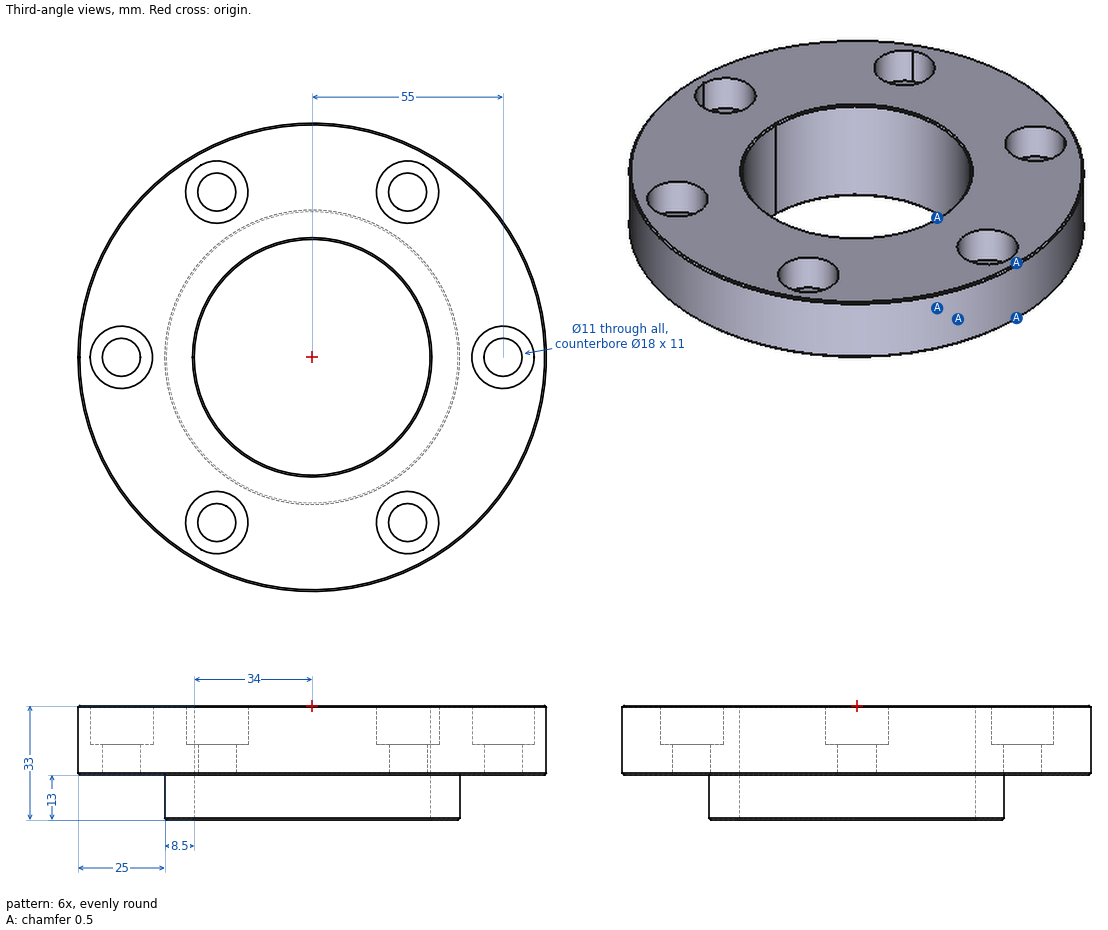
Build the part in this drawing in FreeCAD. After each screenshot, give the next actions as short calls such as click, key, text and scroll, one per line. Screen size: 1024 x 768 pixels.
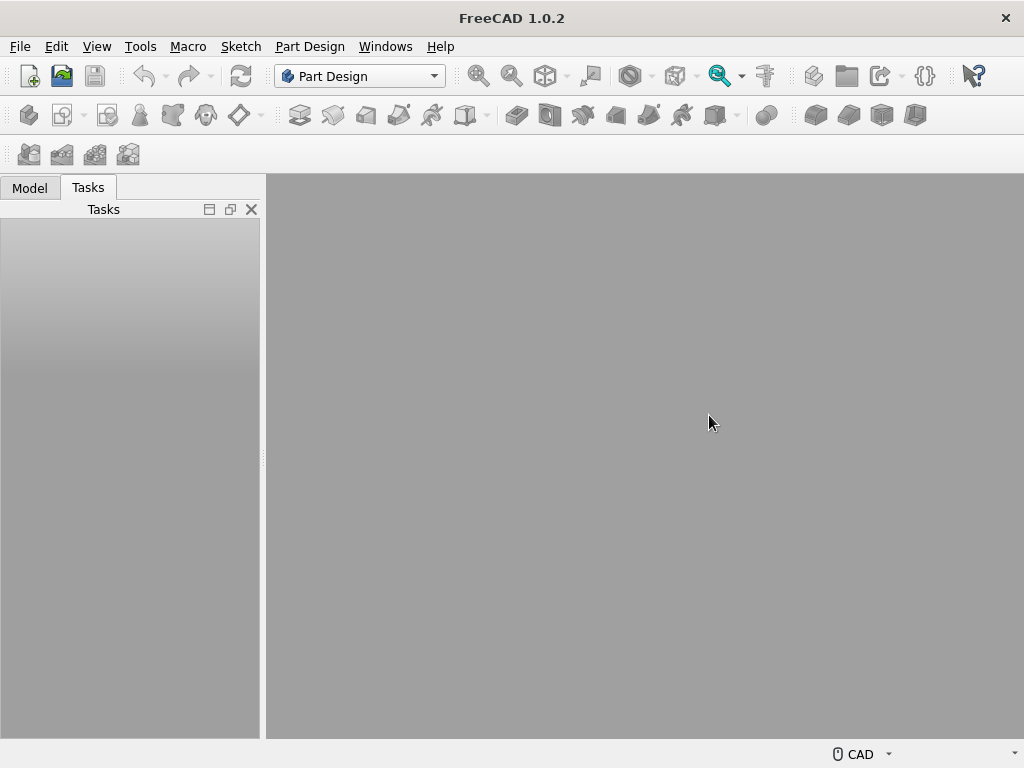
click(29, 76)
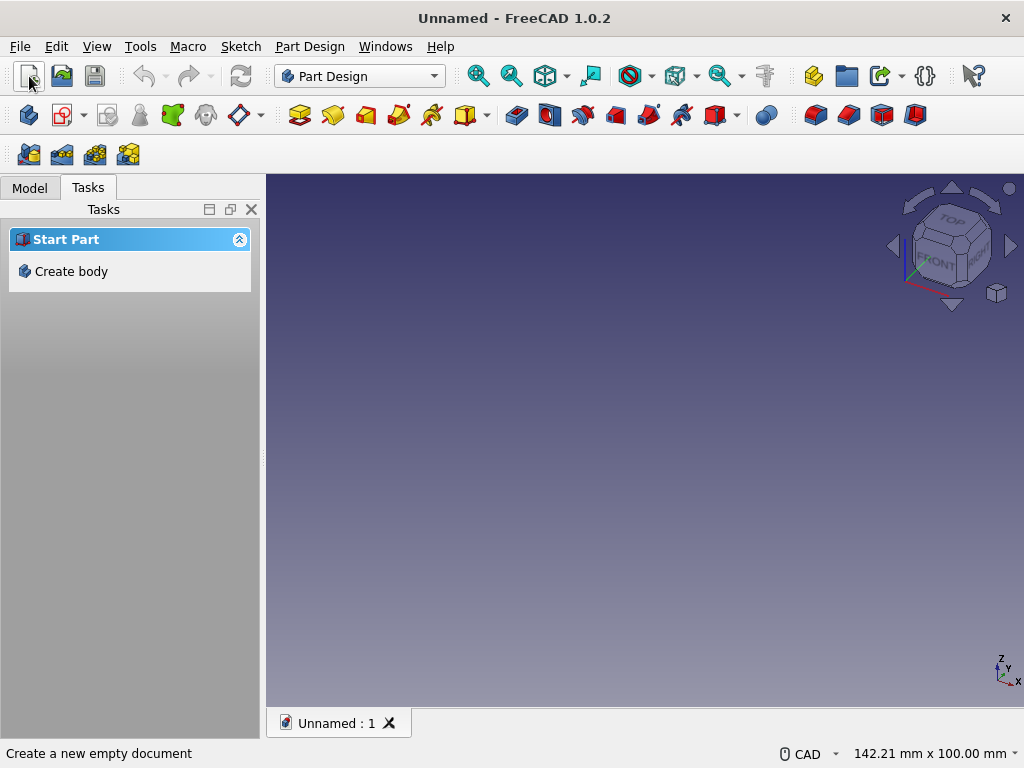
click(62, 116)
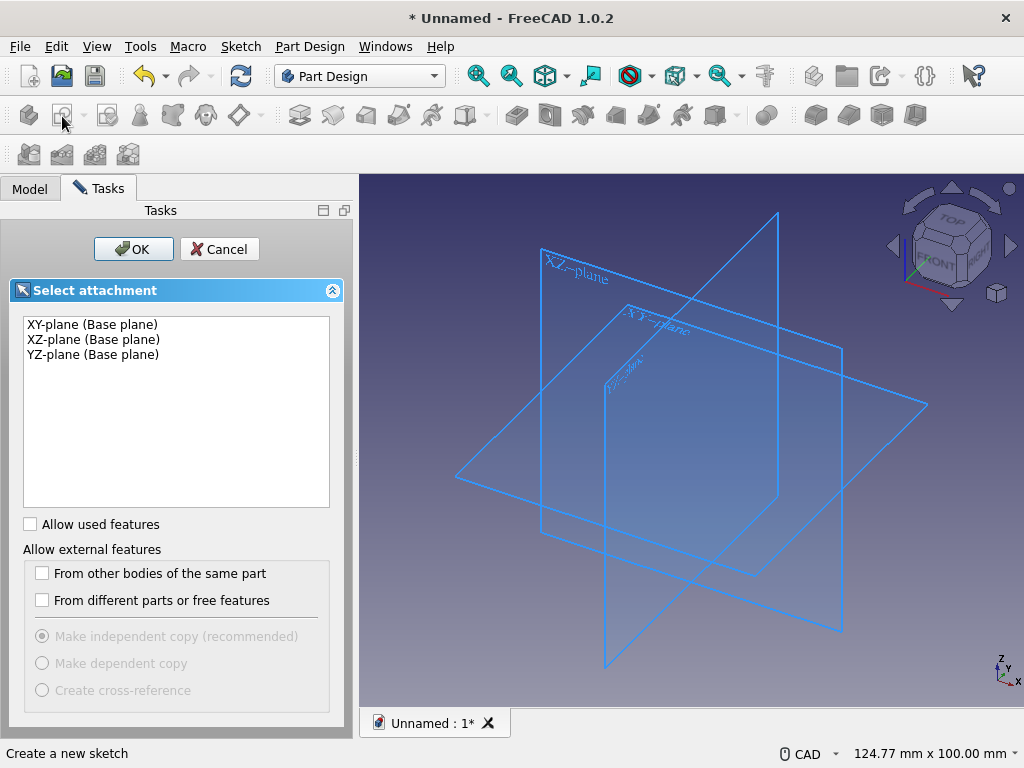
click(84, 340)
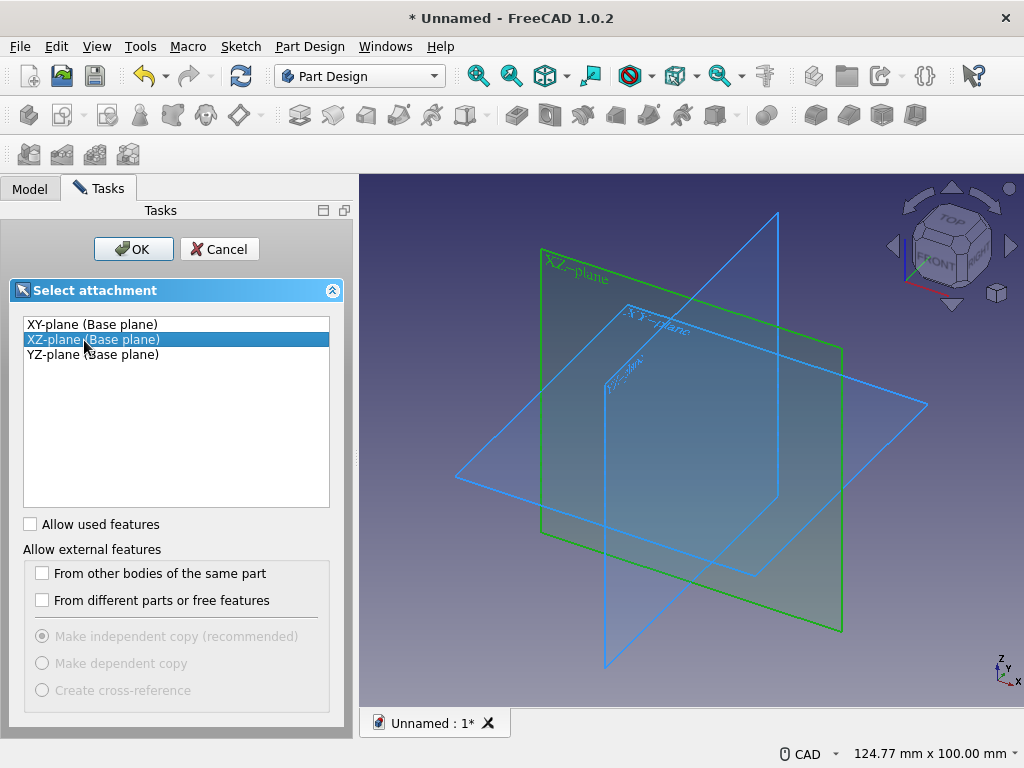
click(134, 249)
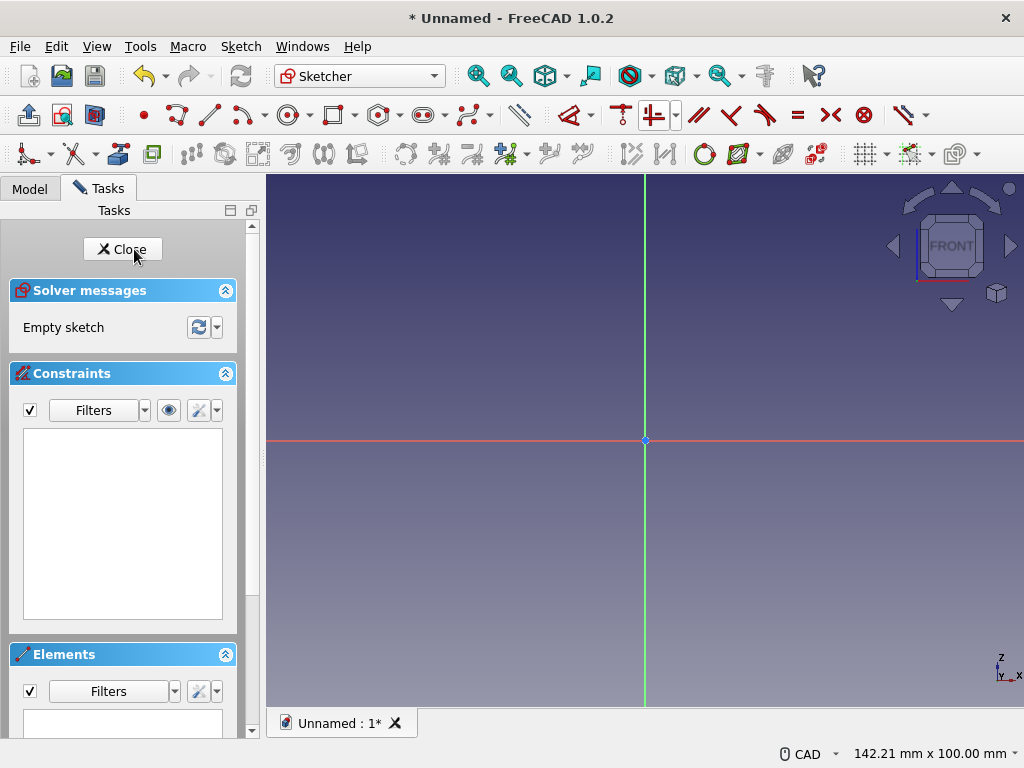
scroll(859, 202, down, 1)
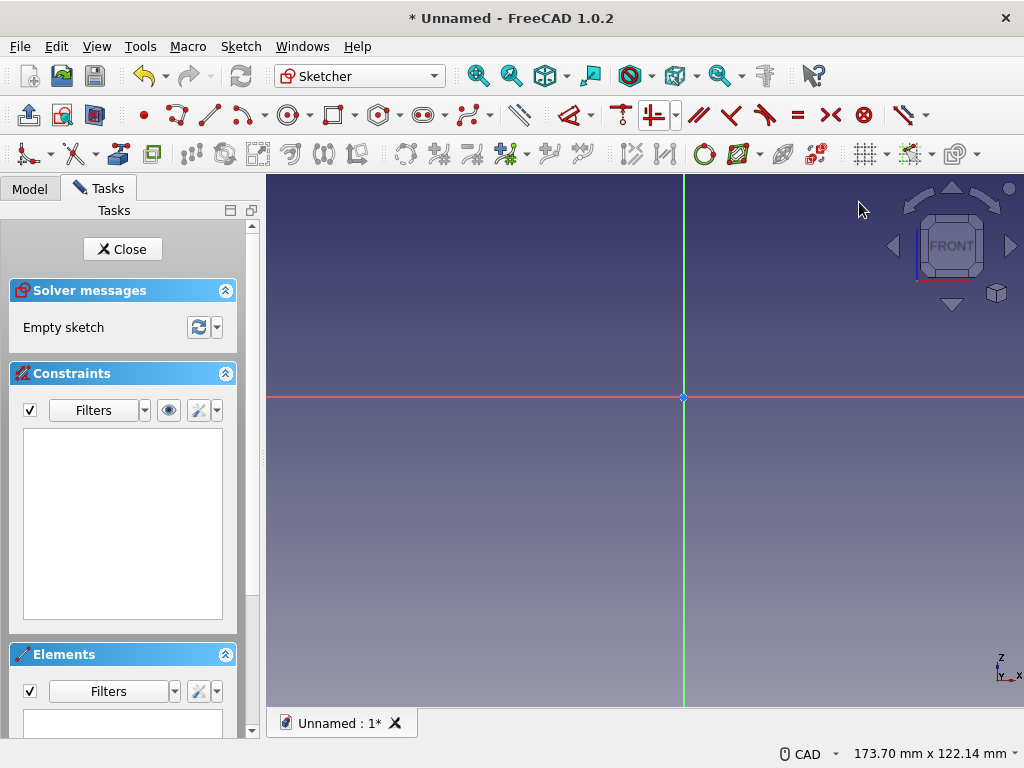
scroll(456, 528, up, 2)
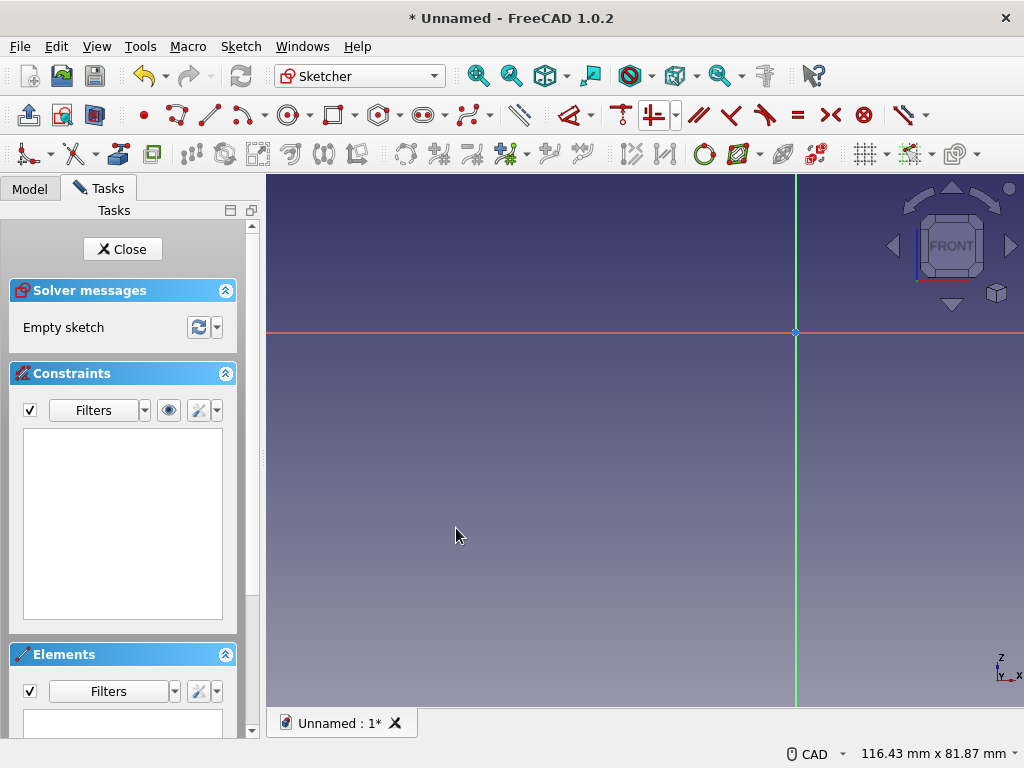
click(177, 116)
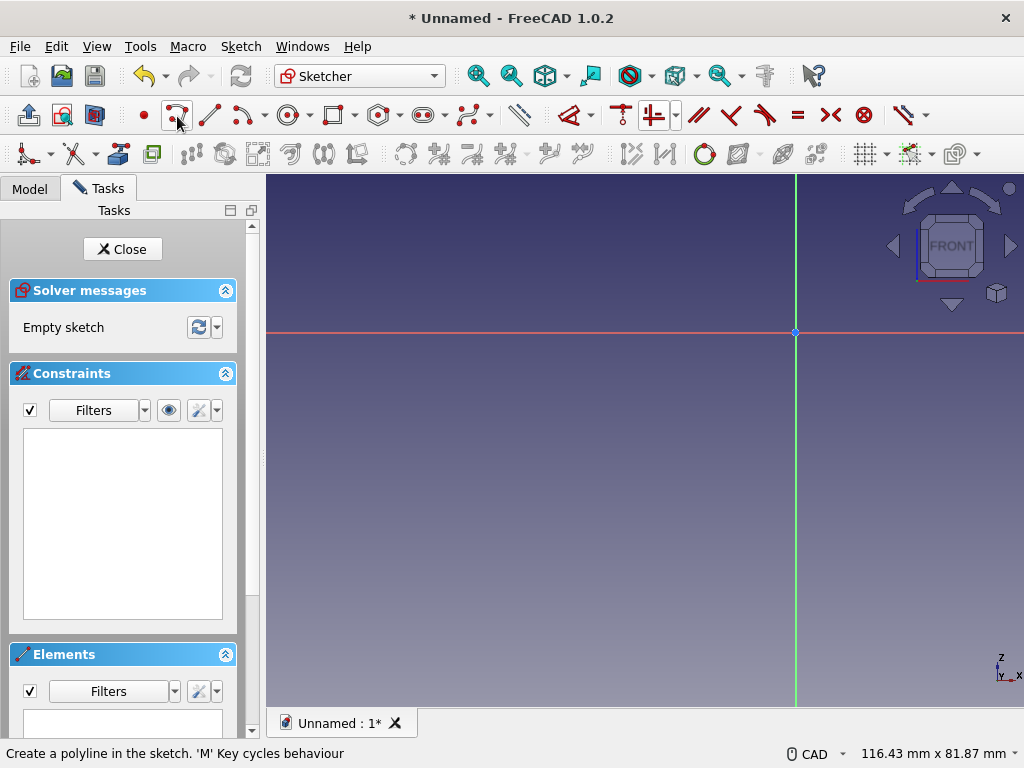
click(575, 333)
click(575, 547)
click(519, 547)
click(519, 463)
click(356, 463)
click(356, 342)
click(575, 333)
key(Escape)
key(Escape)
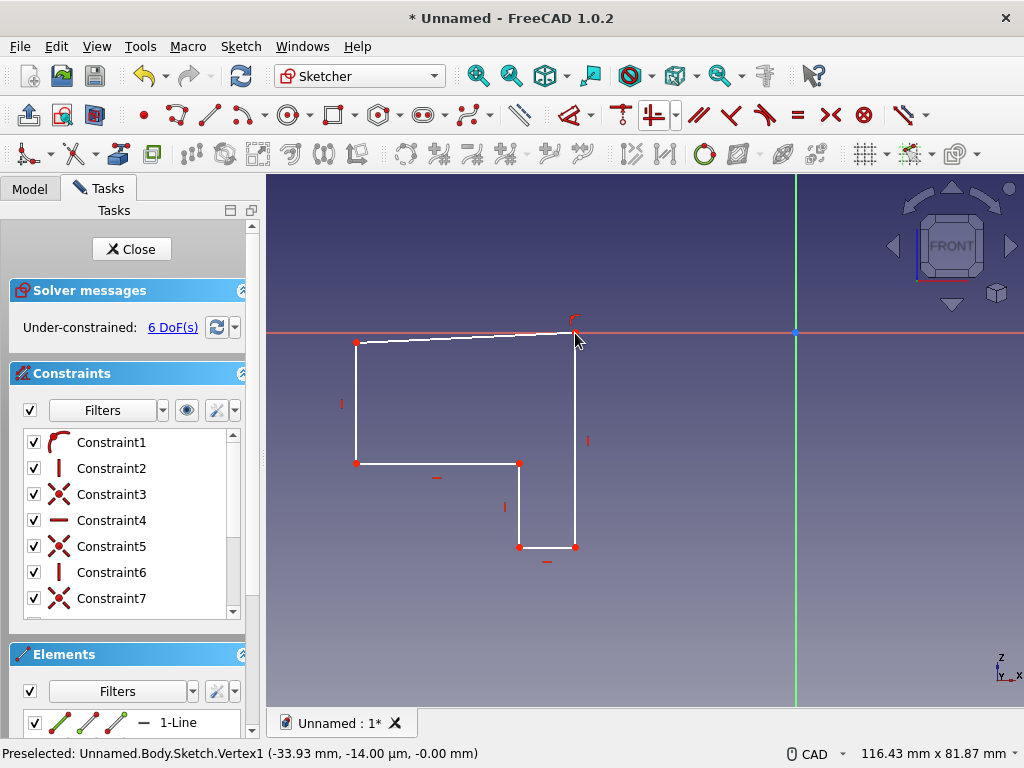
click(509, 336)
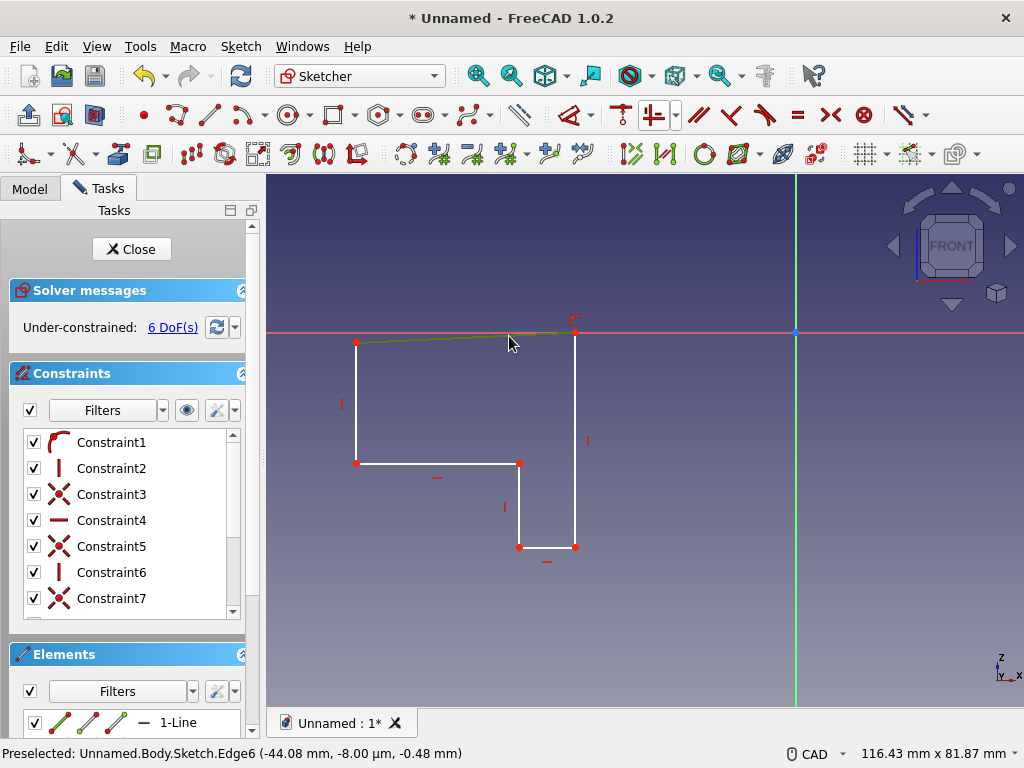
click(676, 116)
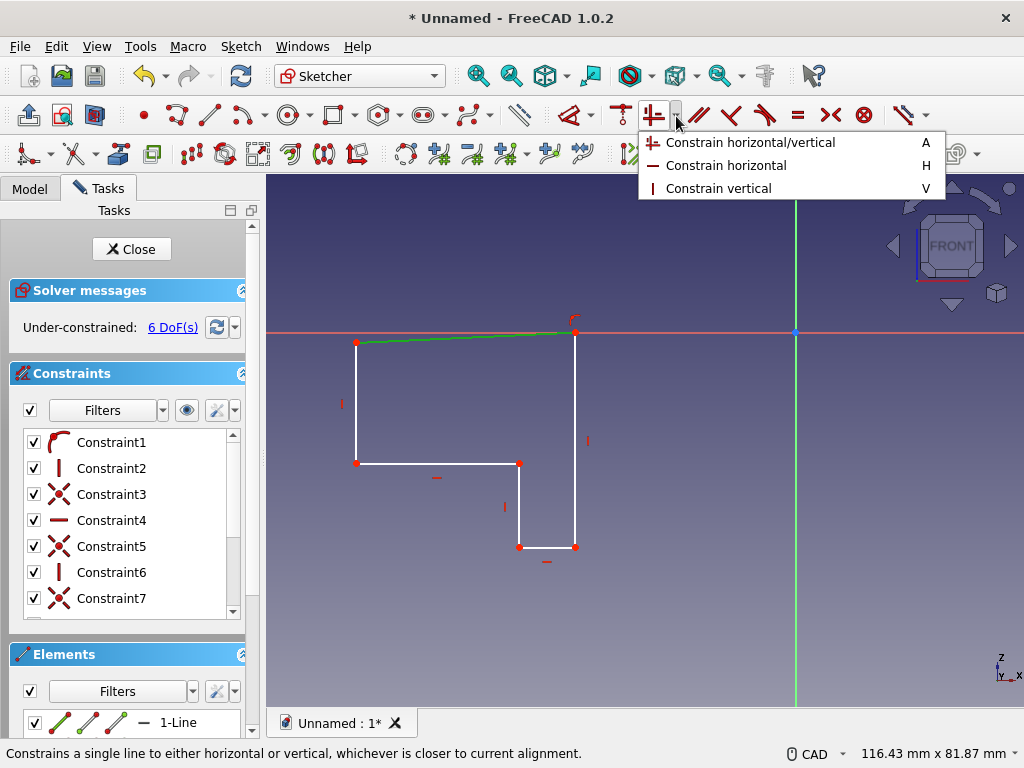
click(792, 166)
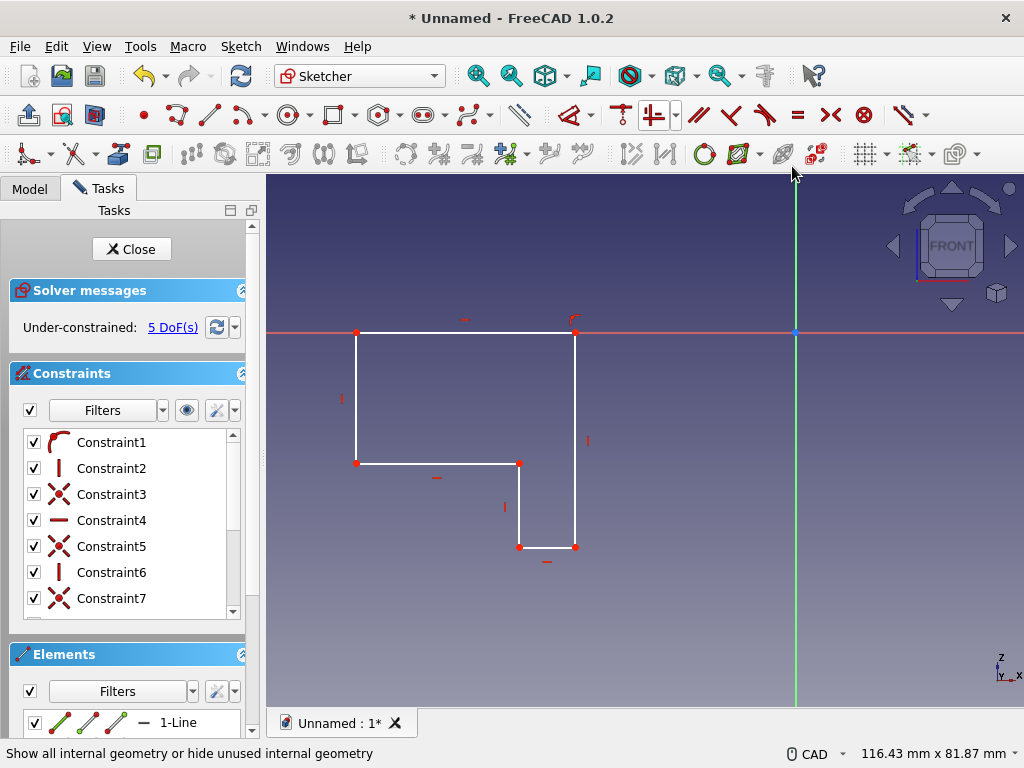
click(568, 116)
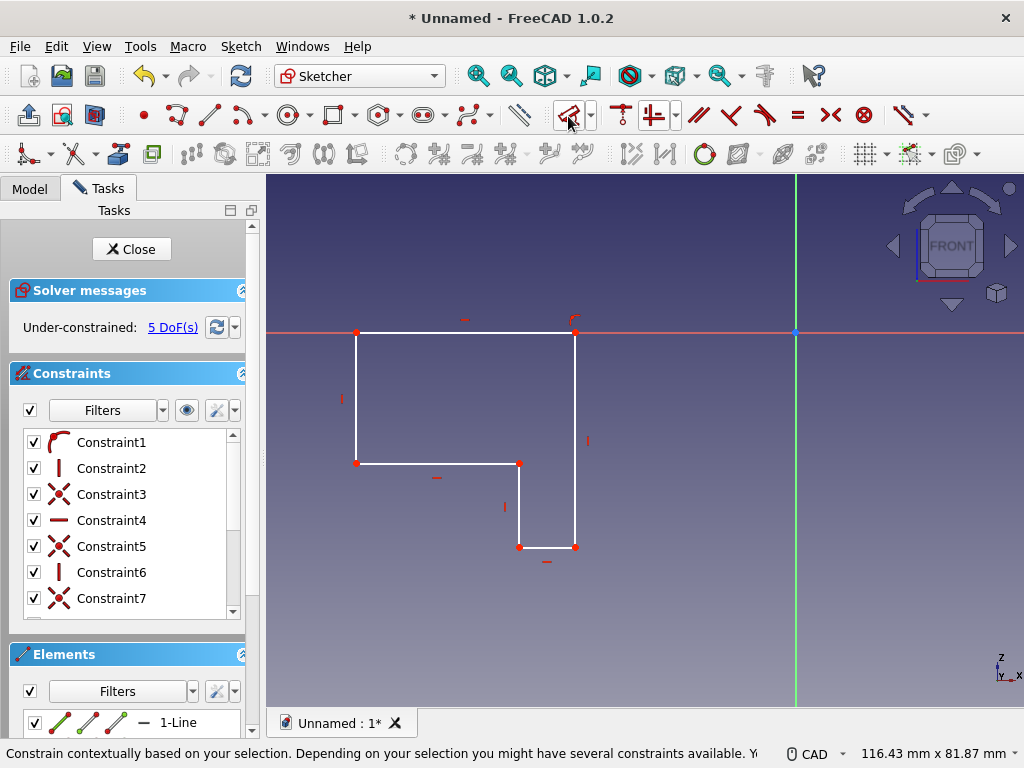
click(575, 397)
click(541, 440)